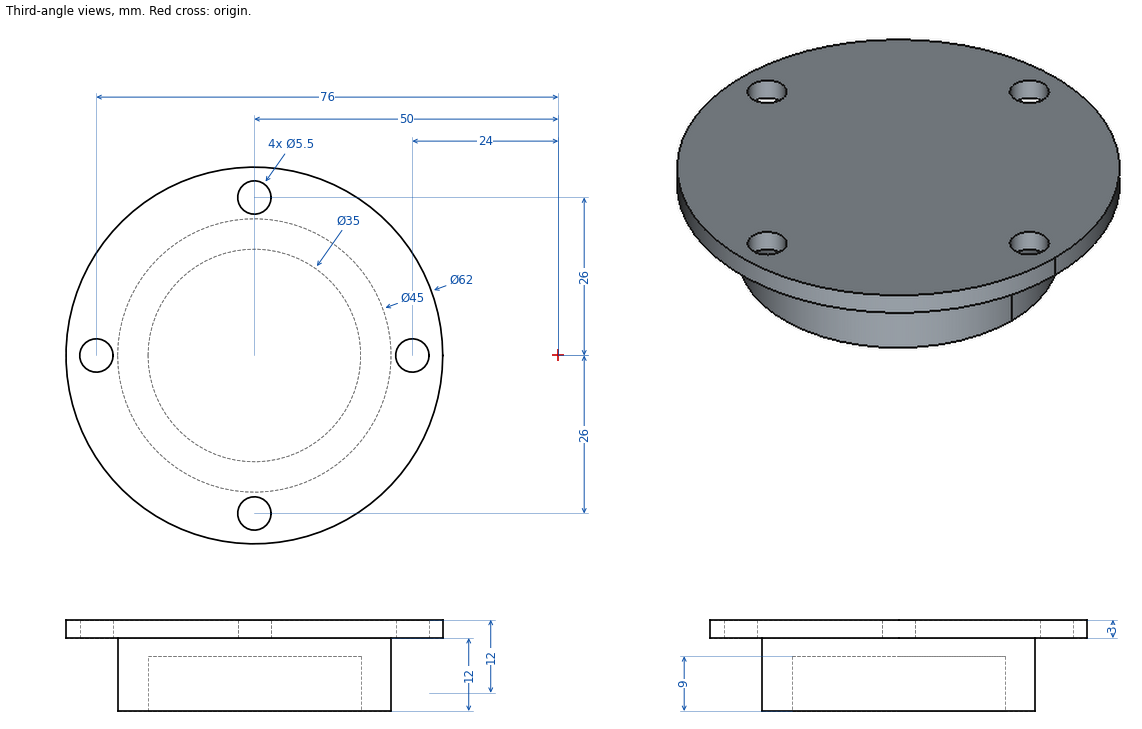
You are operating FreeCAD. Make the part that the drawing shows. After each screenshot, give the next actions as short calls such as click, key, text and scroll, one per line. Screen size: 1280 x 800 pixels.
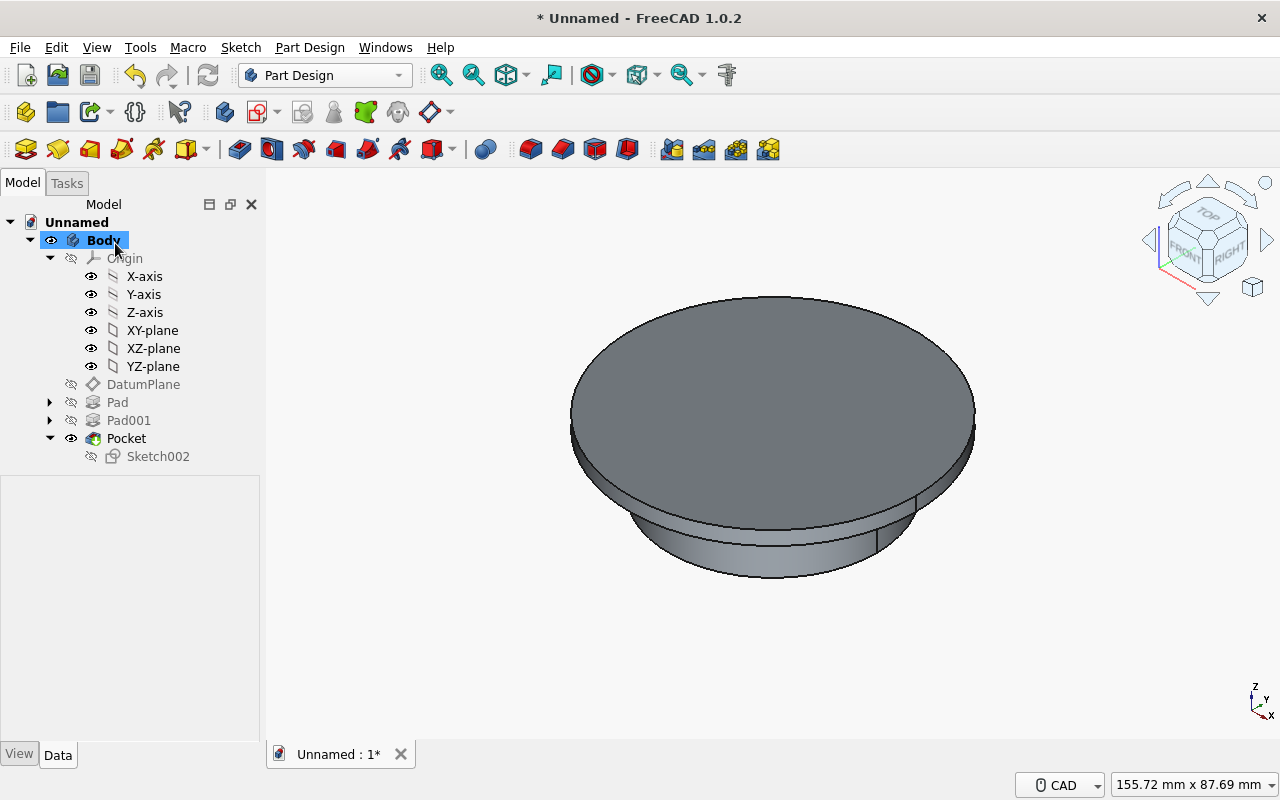
click(773, 413)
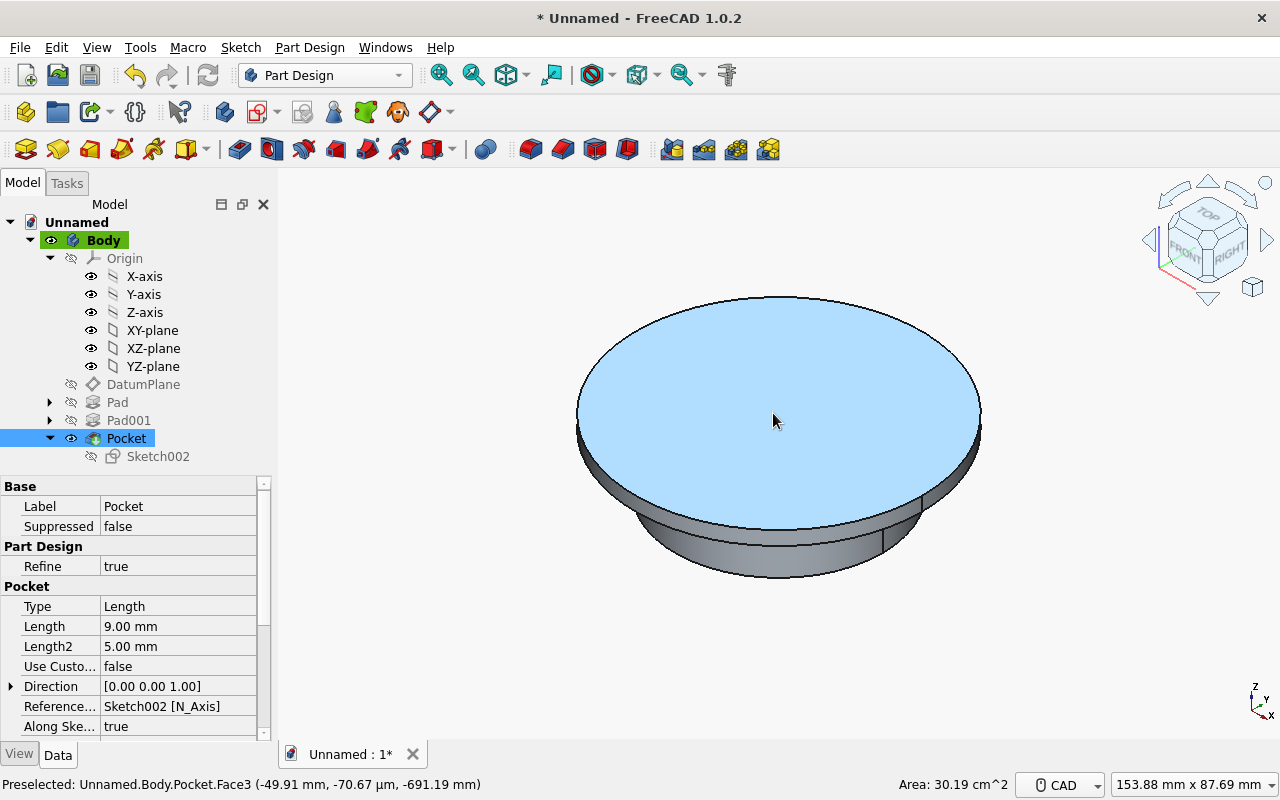
click(258, 112)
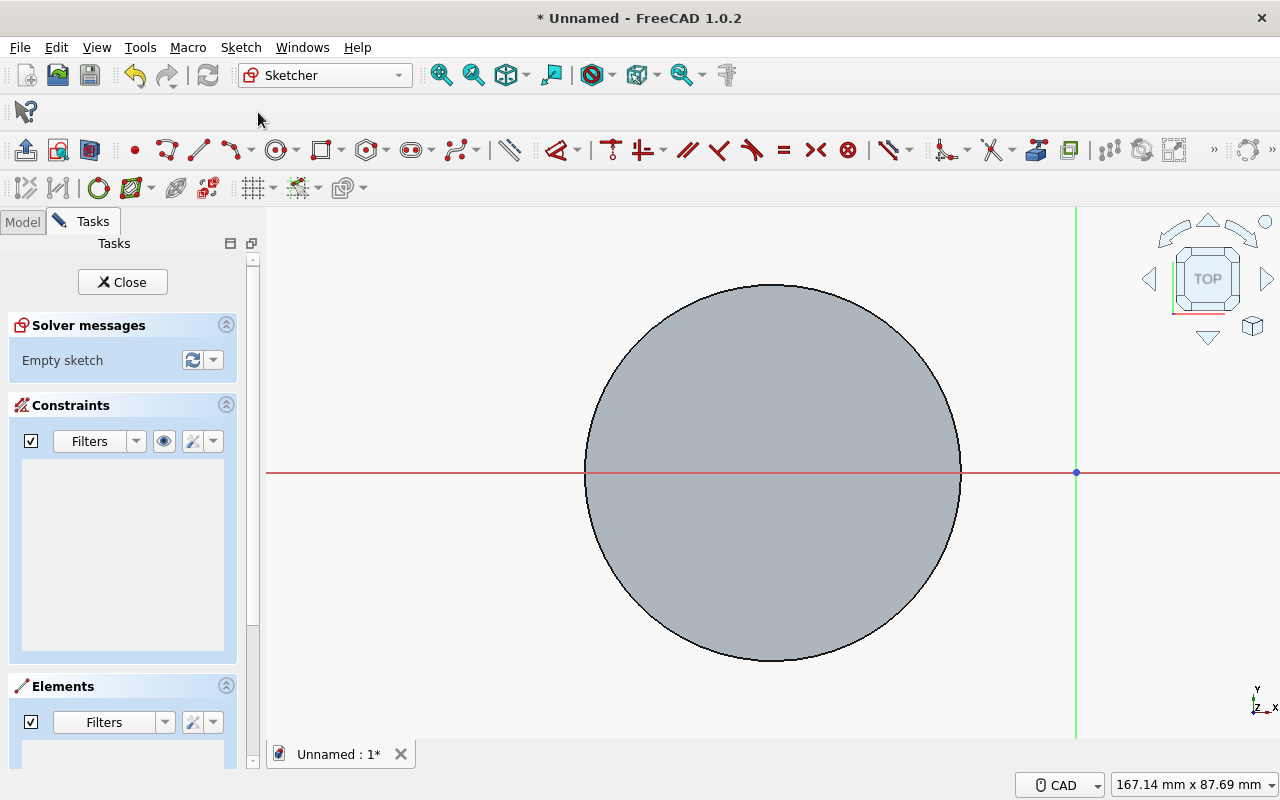
click(276, 150)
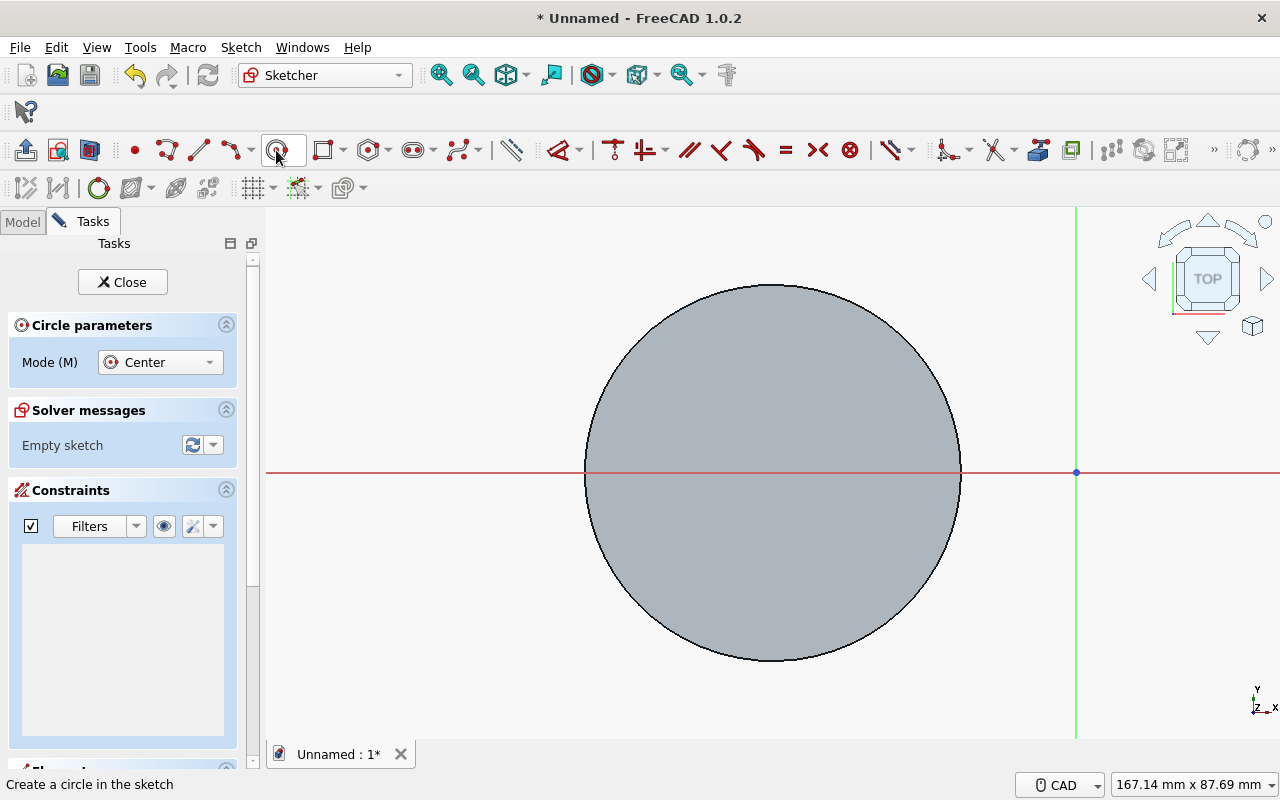
scroll(773, 315, up, 2)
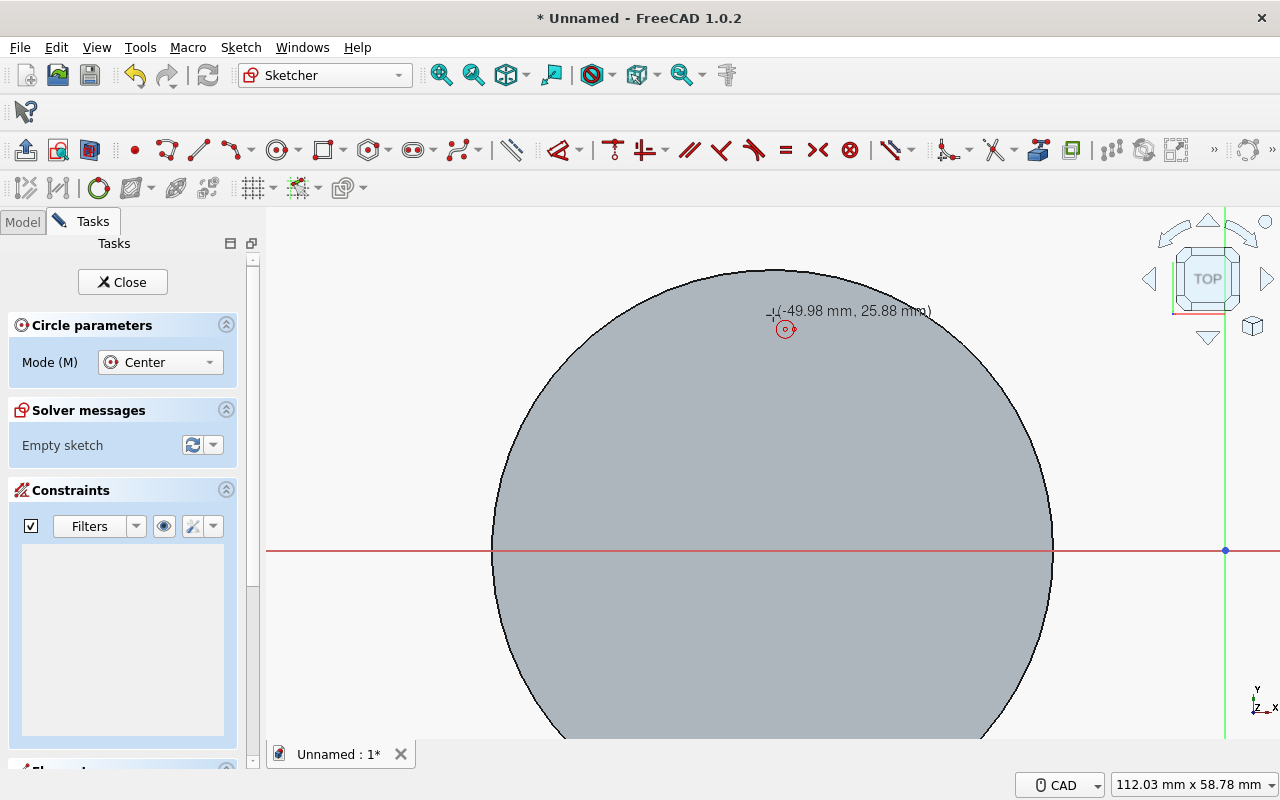
click(773, 315)
move(790, 298)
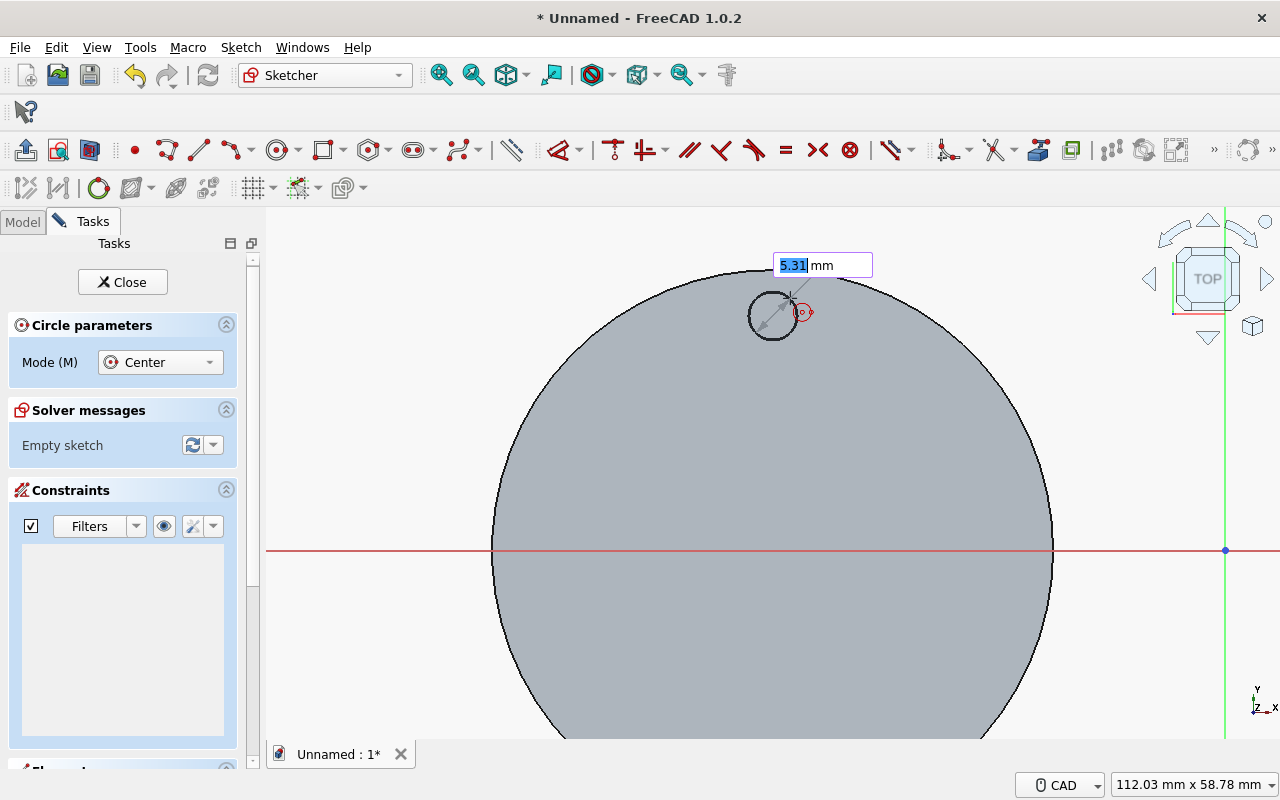
text(5.5)
key(Return)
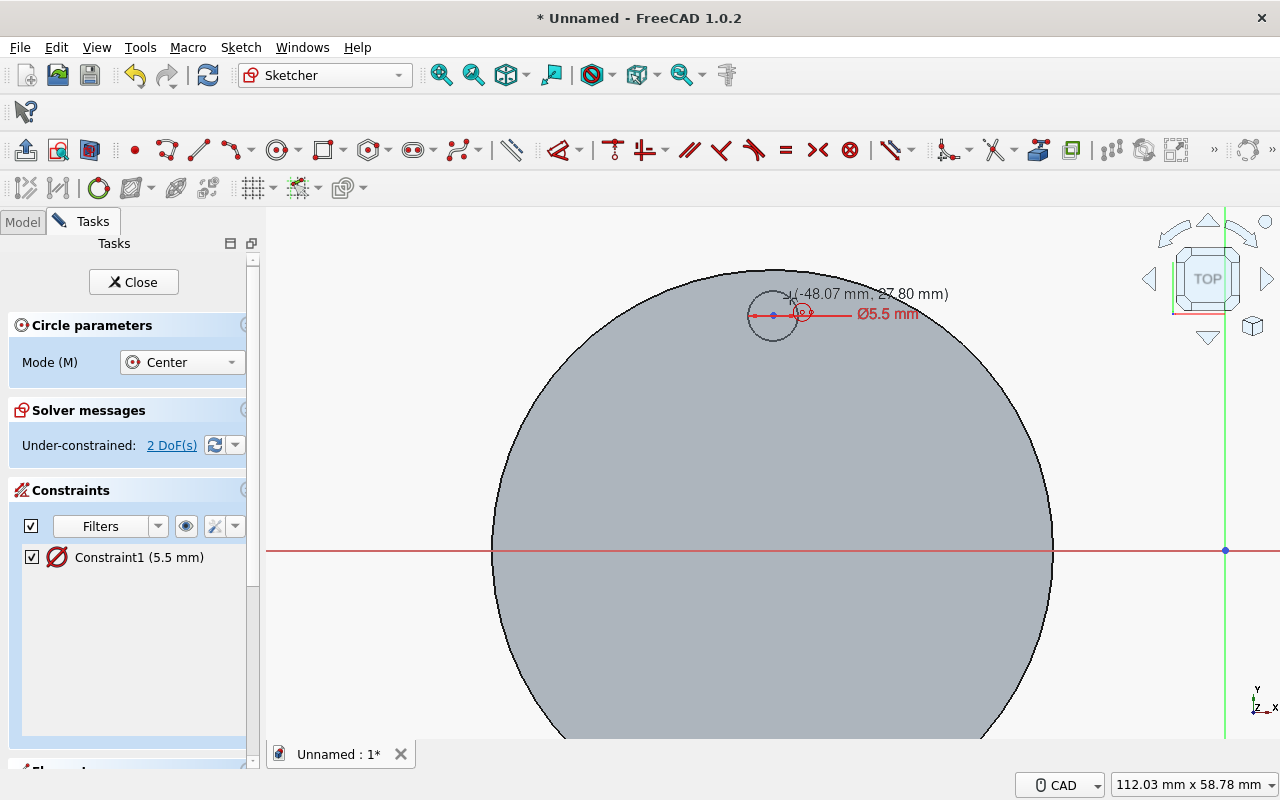
click(1008, 551)
move(1025, 533)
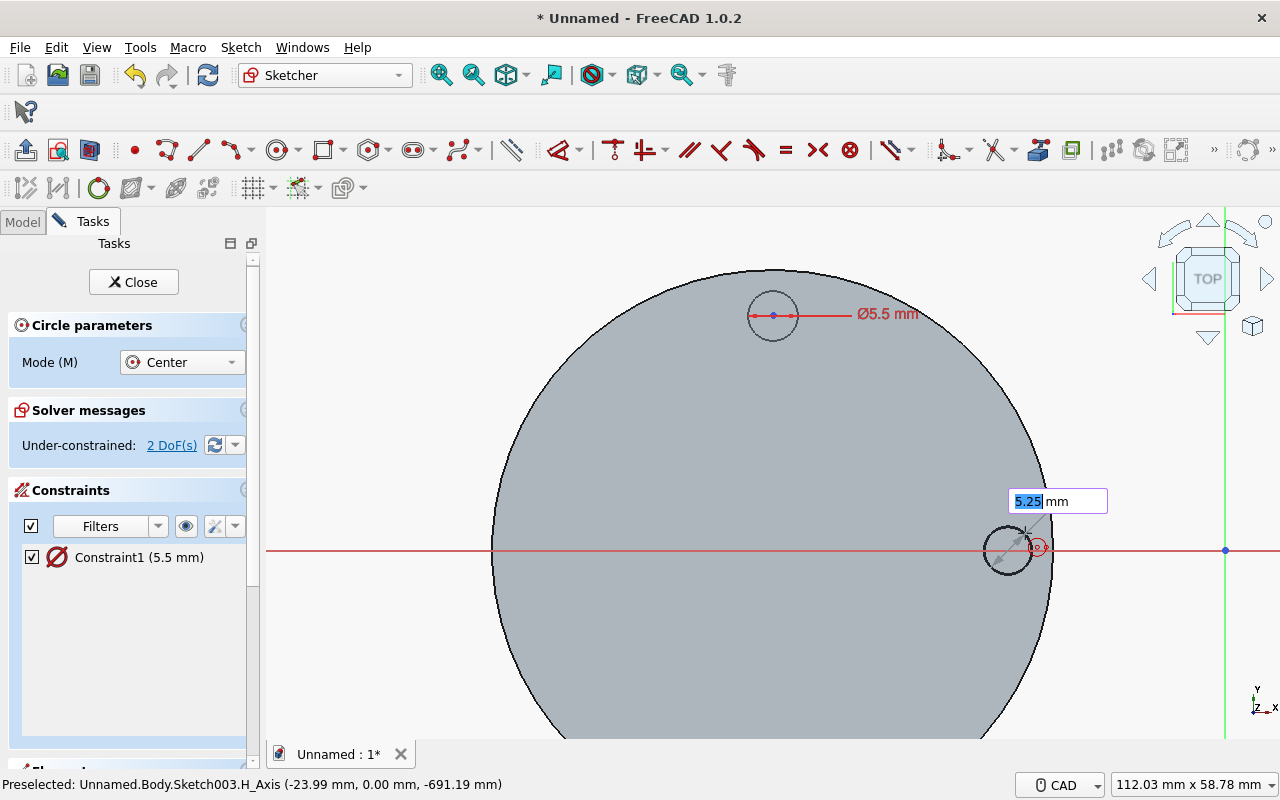
text(5.5)
key(Return)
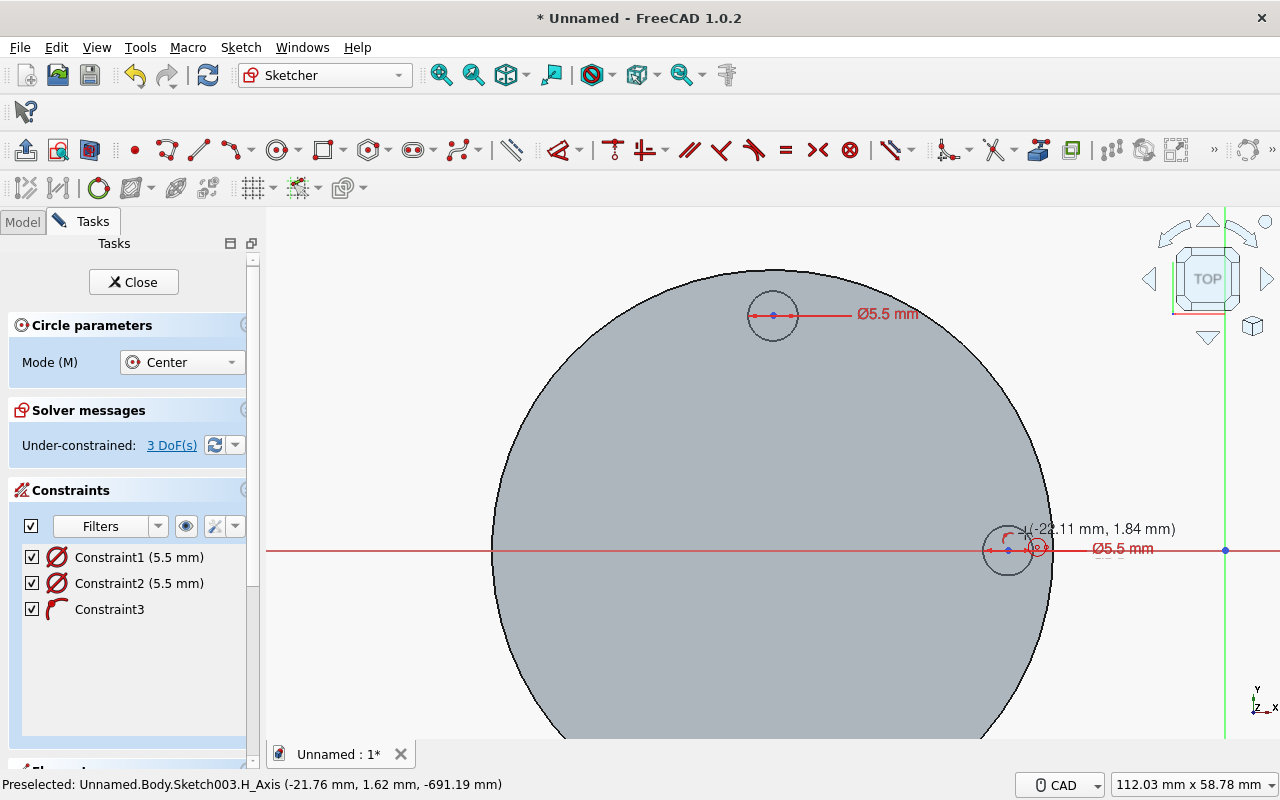
scroll(371, 315, down, 2)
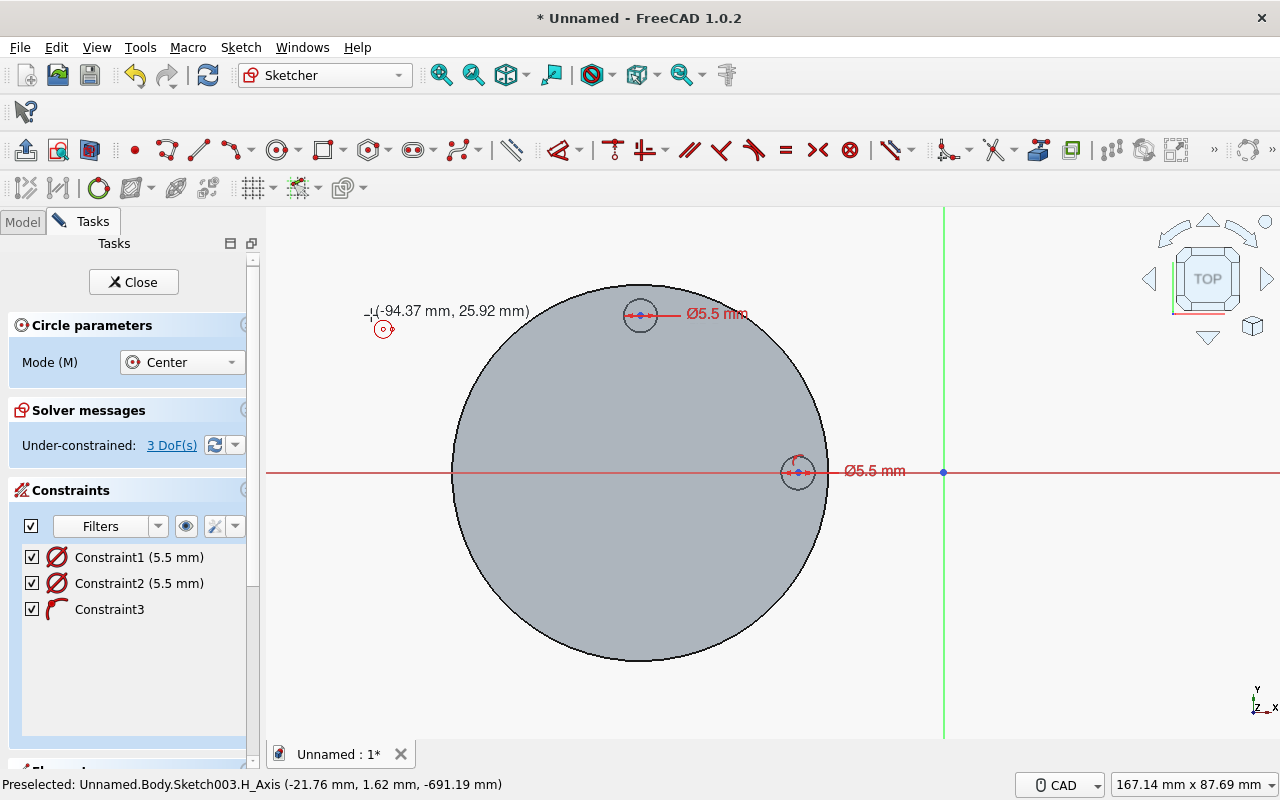
scroll(640, 631, up, 2)